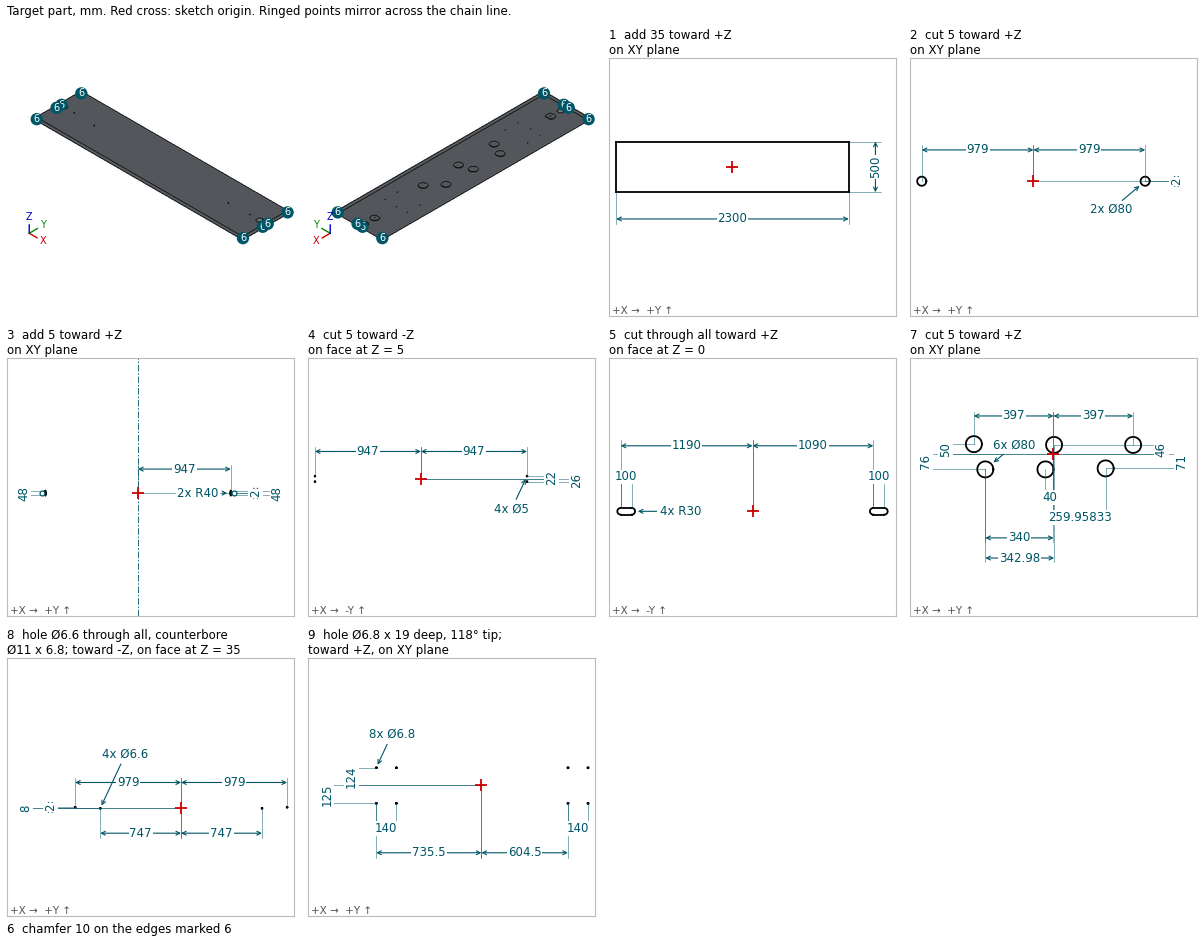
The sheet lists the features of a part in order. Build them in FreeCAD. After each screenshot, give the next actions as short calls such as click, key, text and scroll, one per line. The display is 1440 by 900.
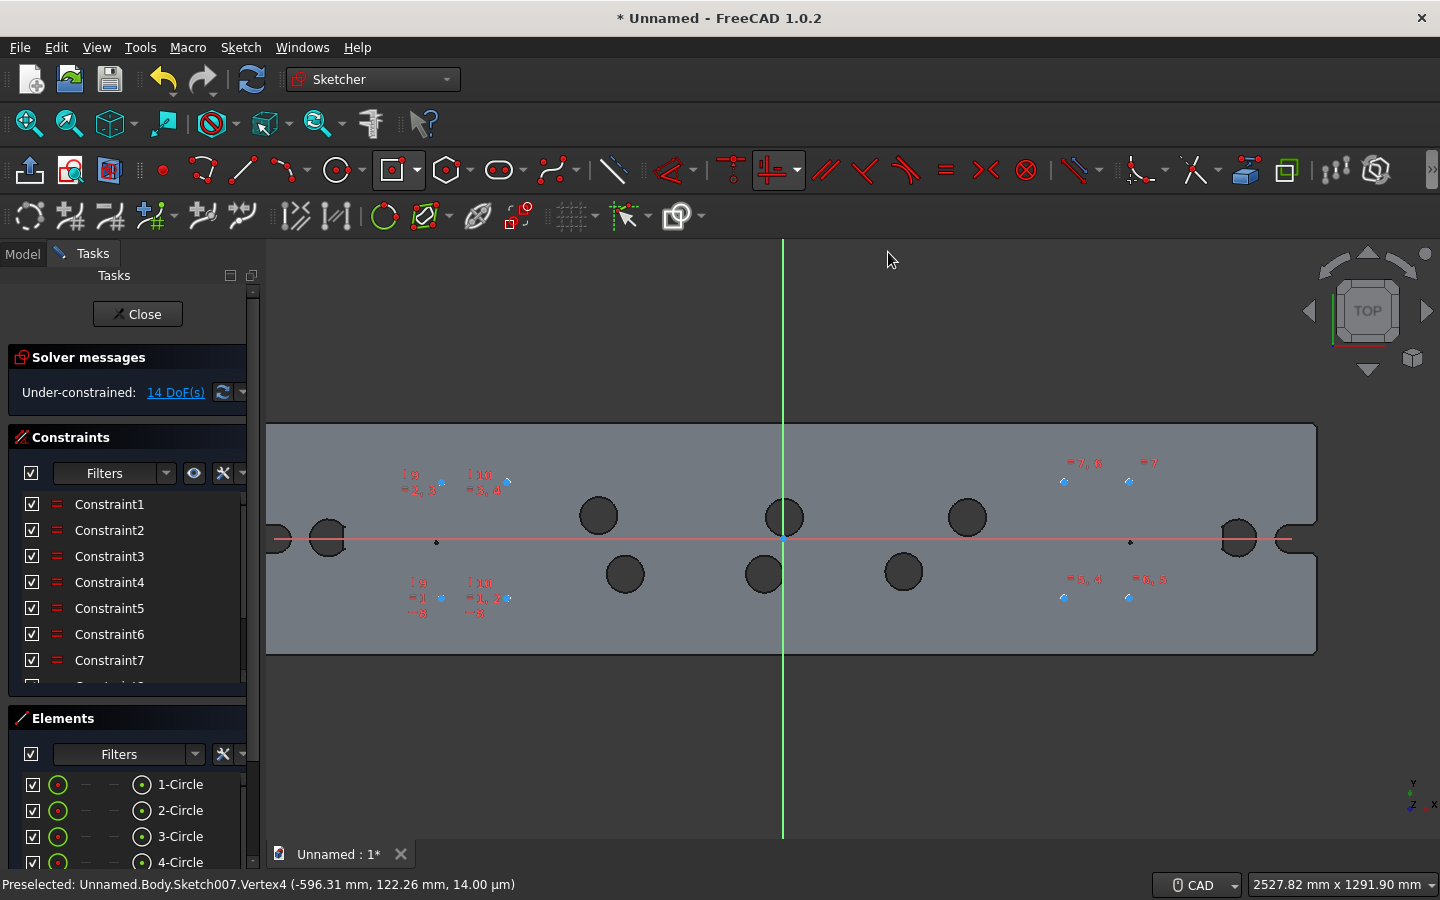
click(441, 483)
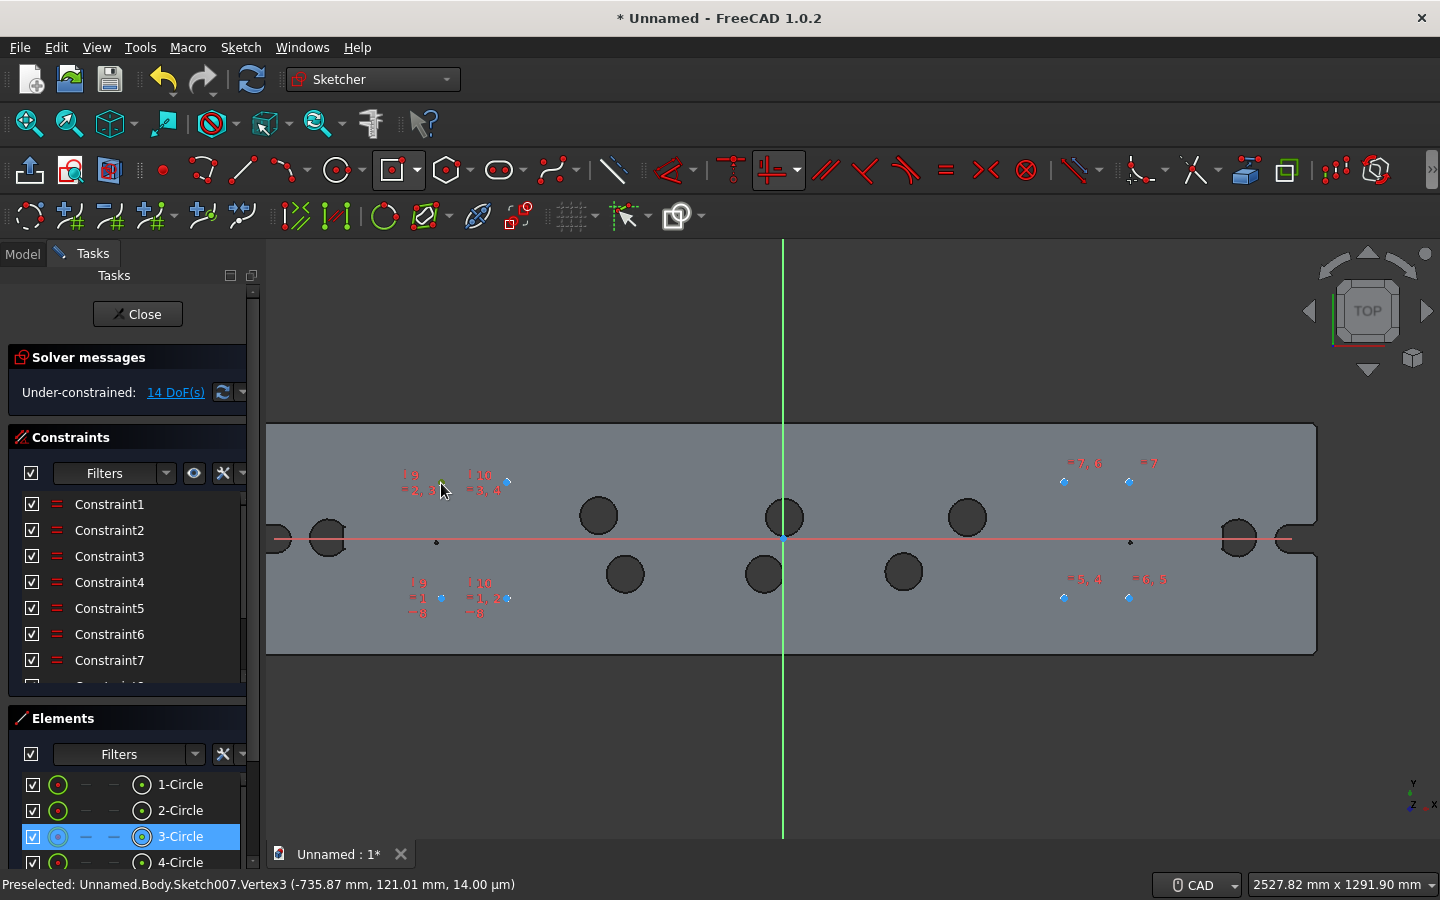
click(507, 482)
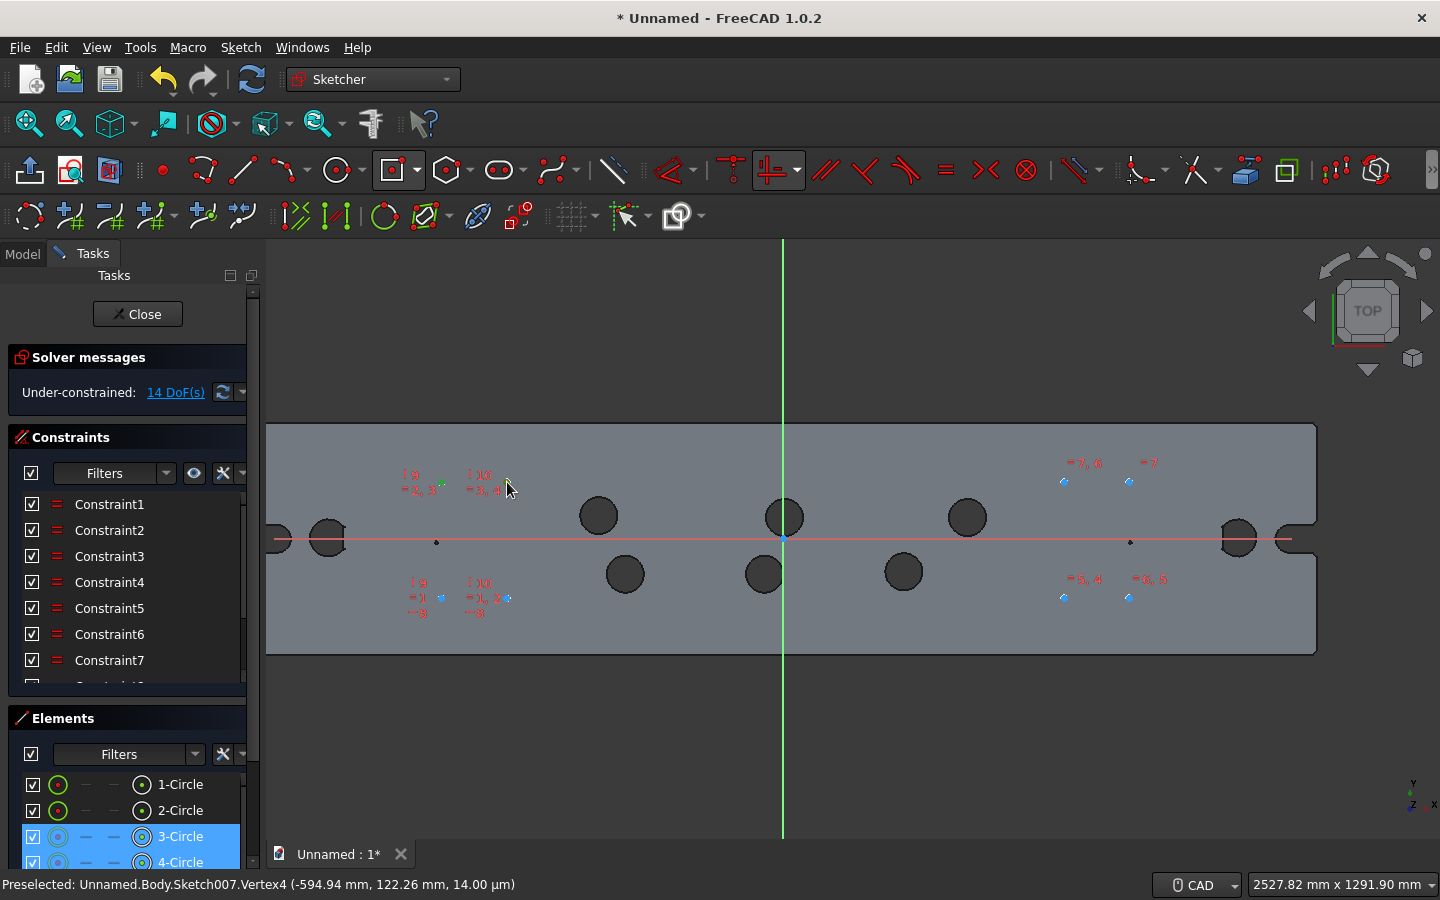
key(h)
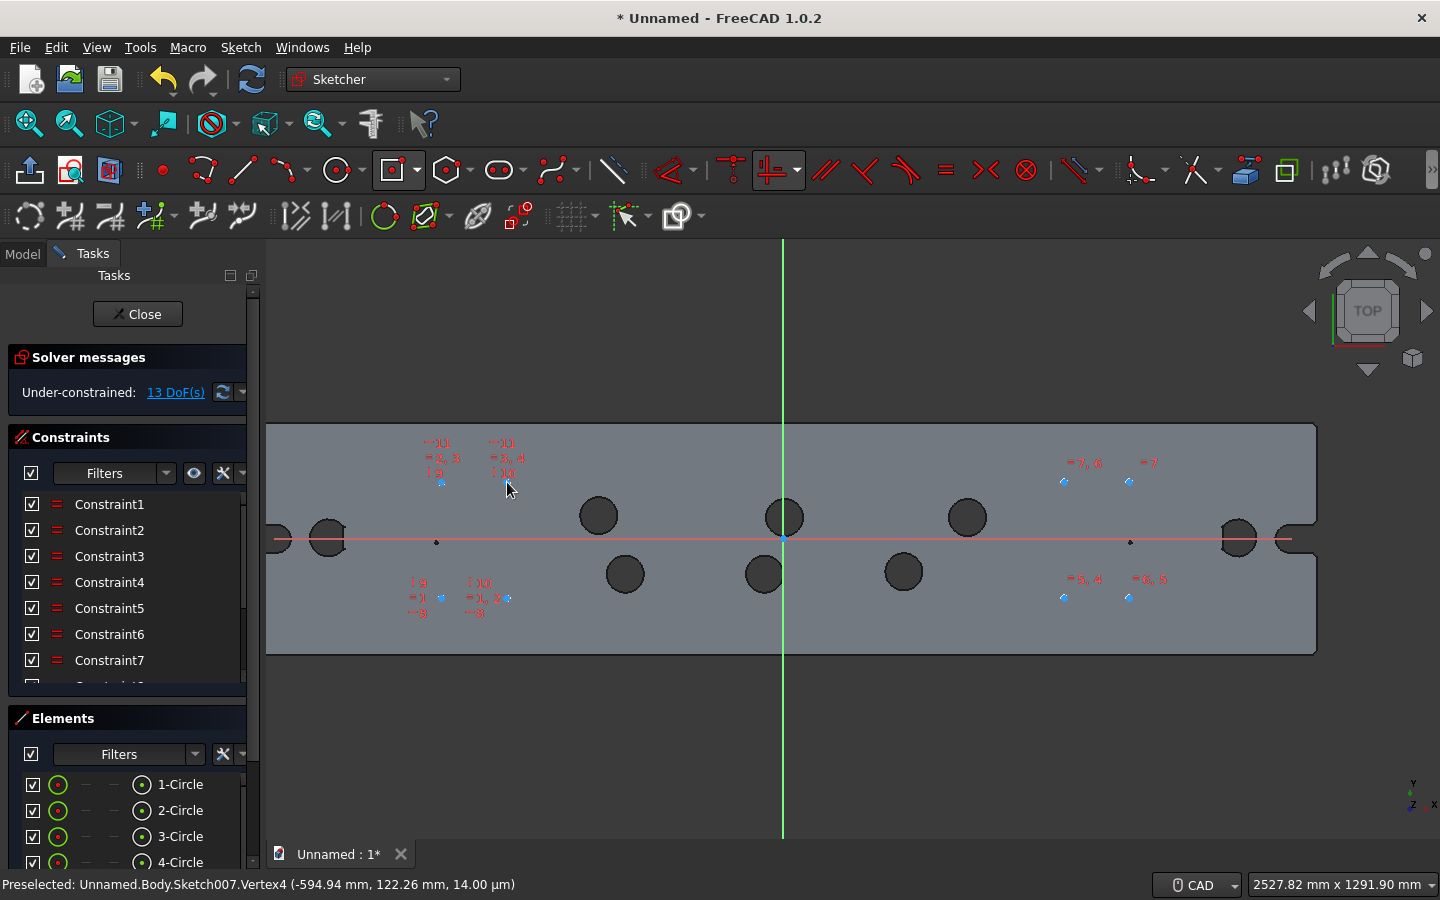
click(507, 598)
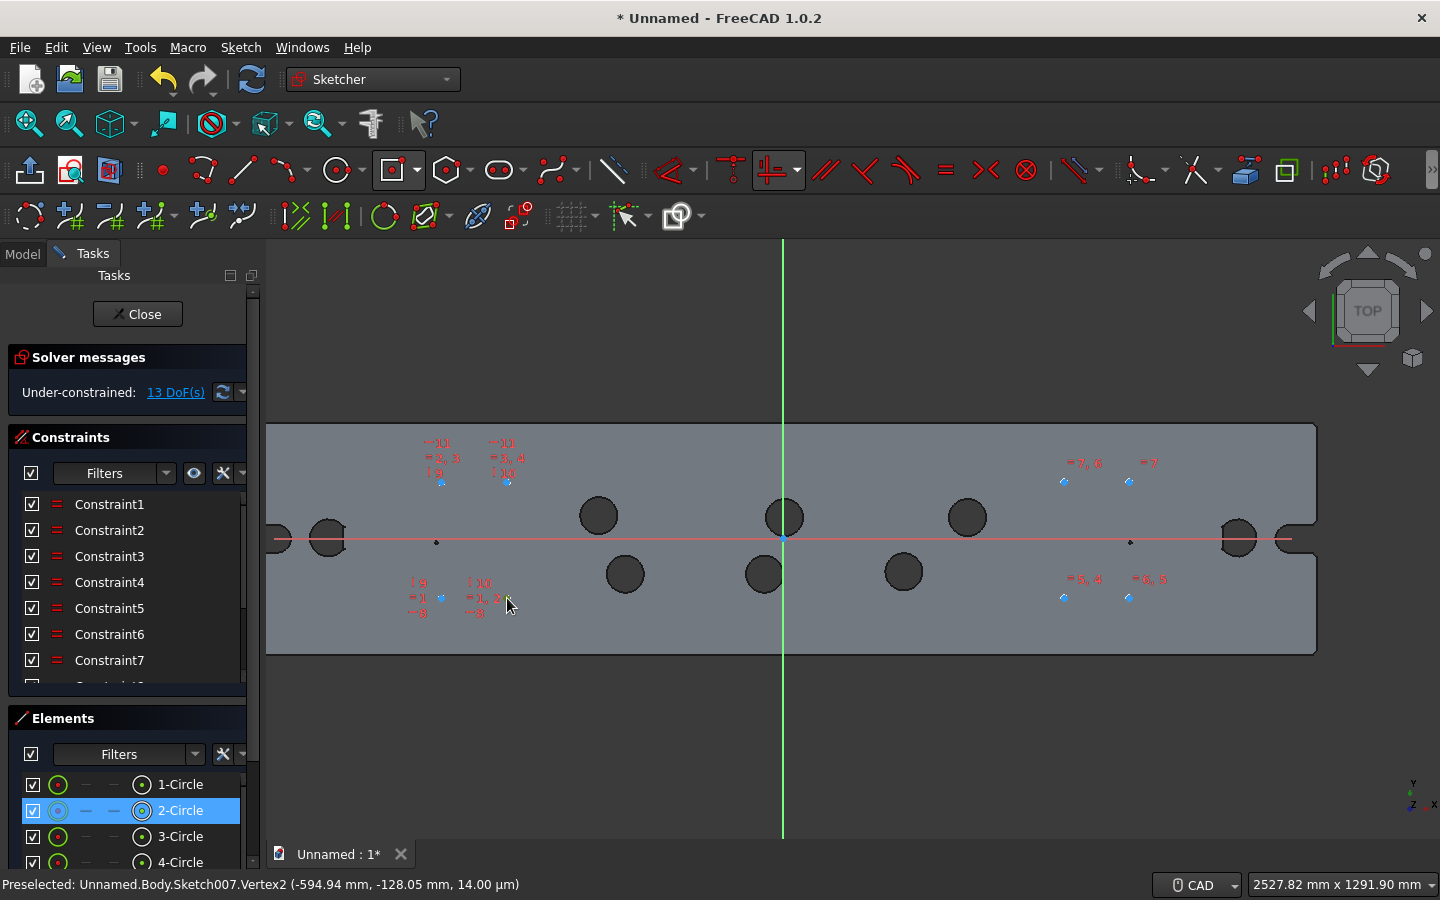
click(1064, 598)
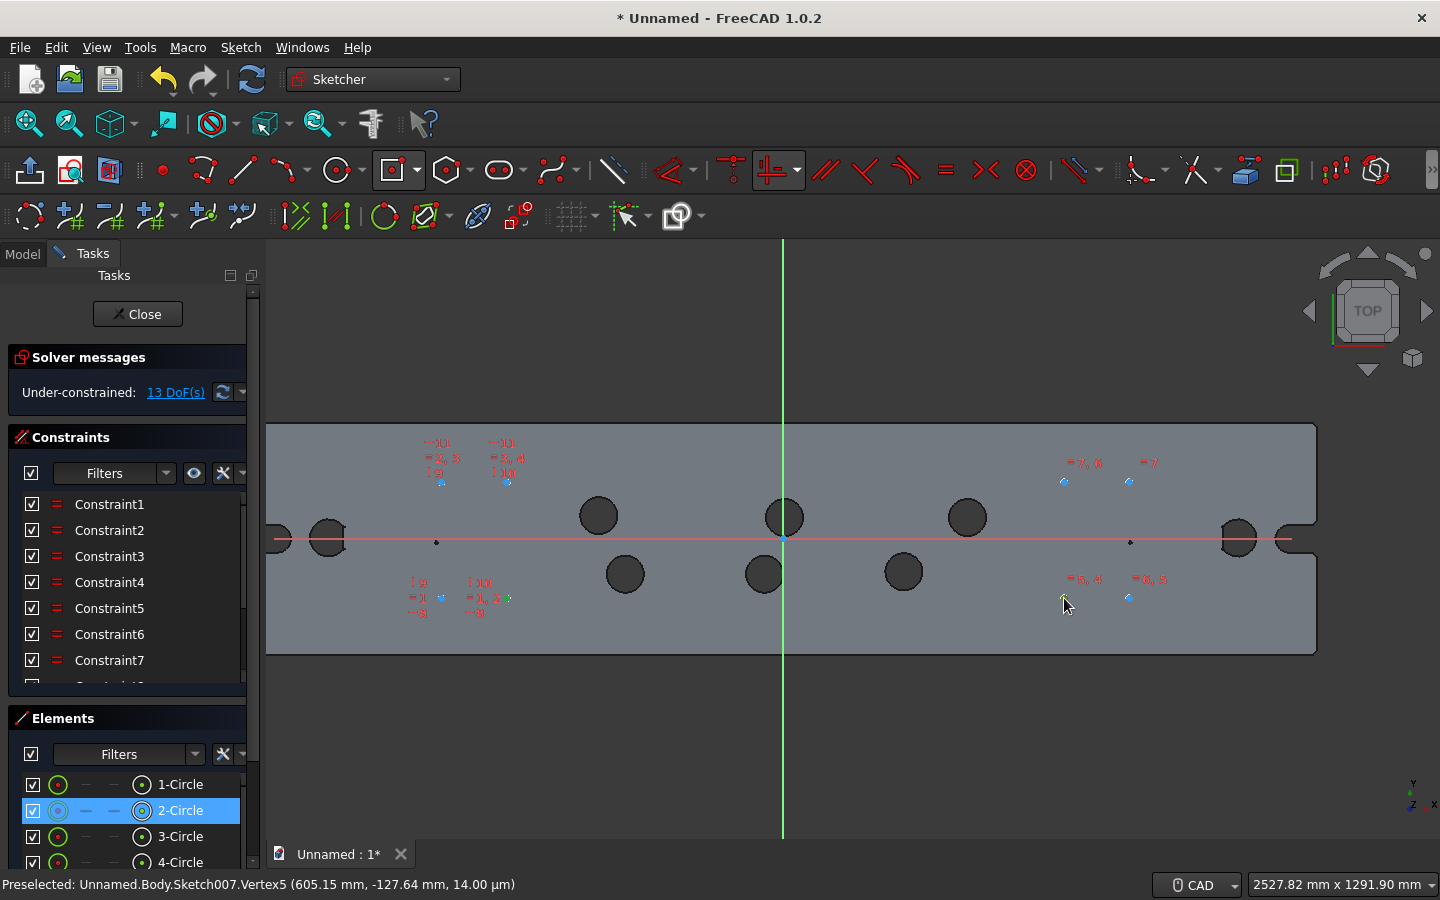
click(800, 170)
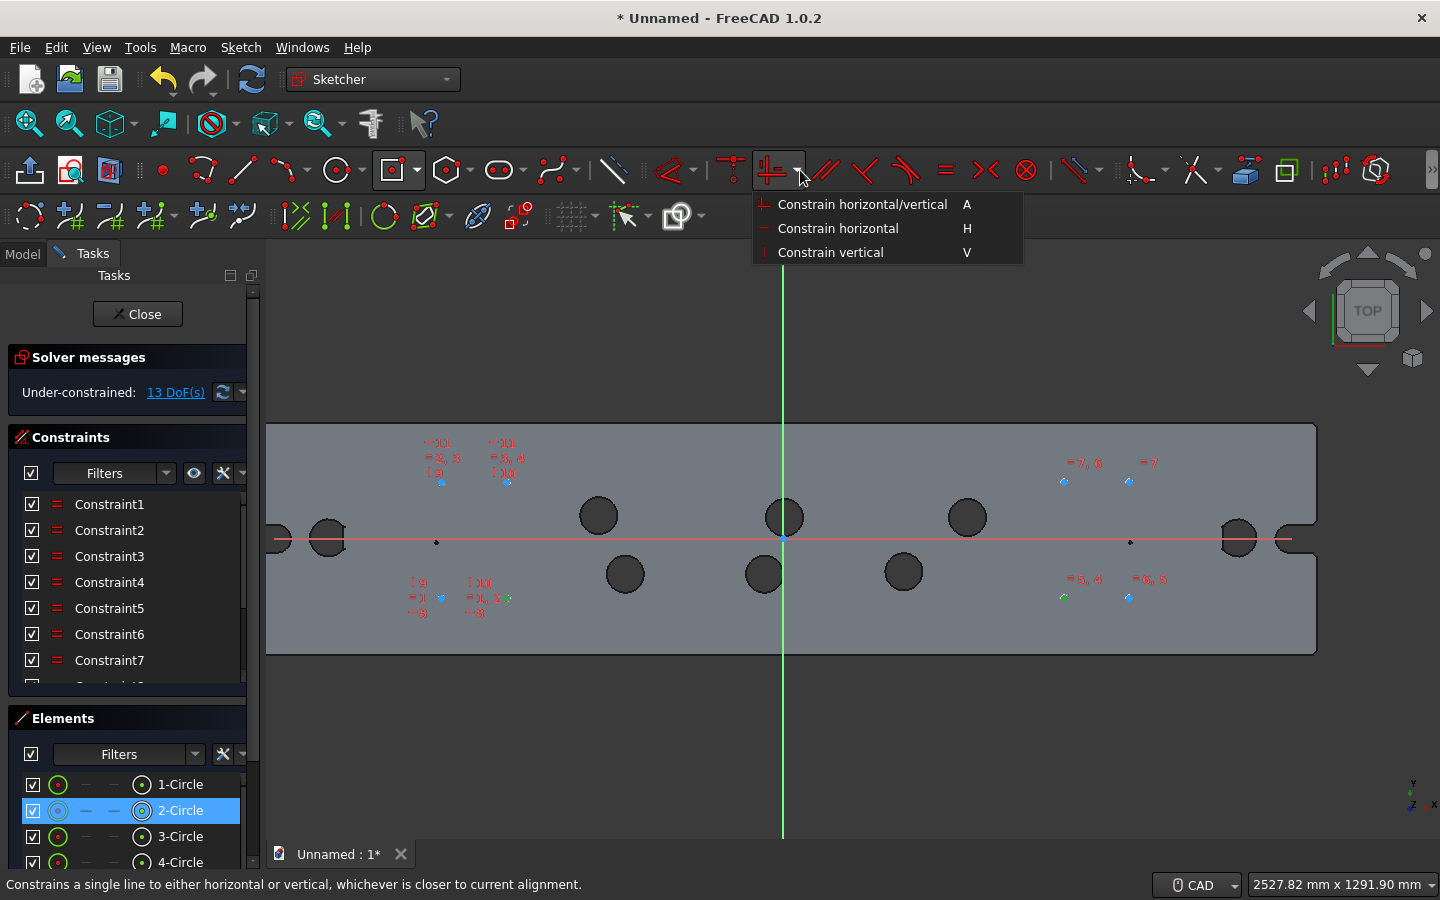
click(888, 228)